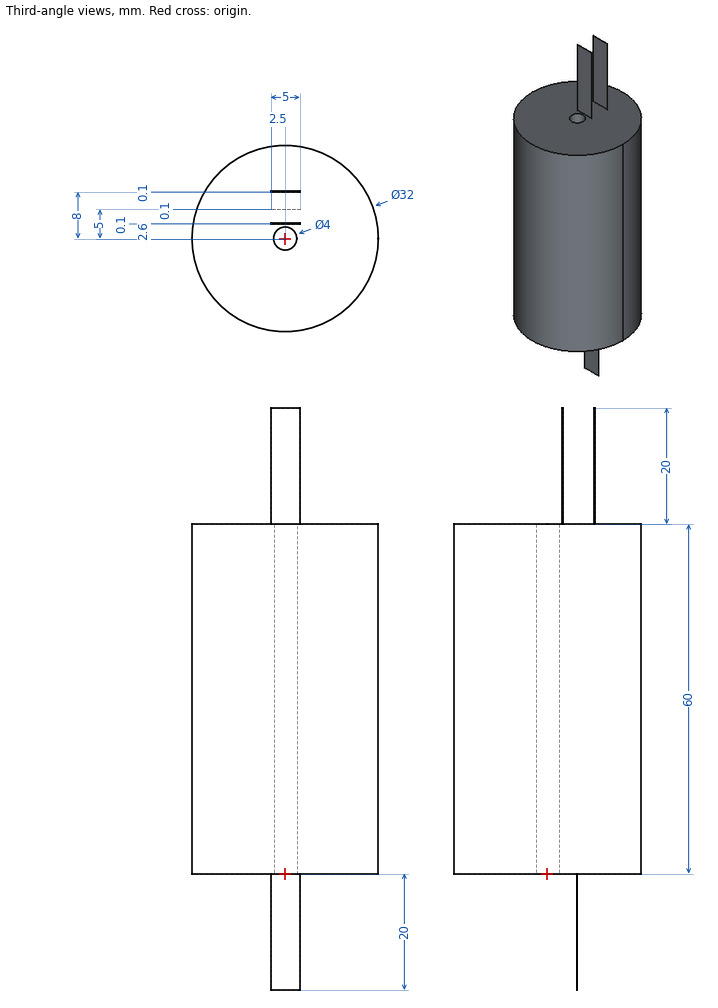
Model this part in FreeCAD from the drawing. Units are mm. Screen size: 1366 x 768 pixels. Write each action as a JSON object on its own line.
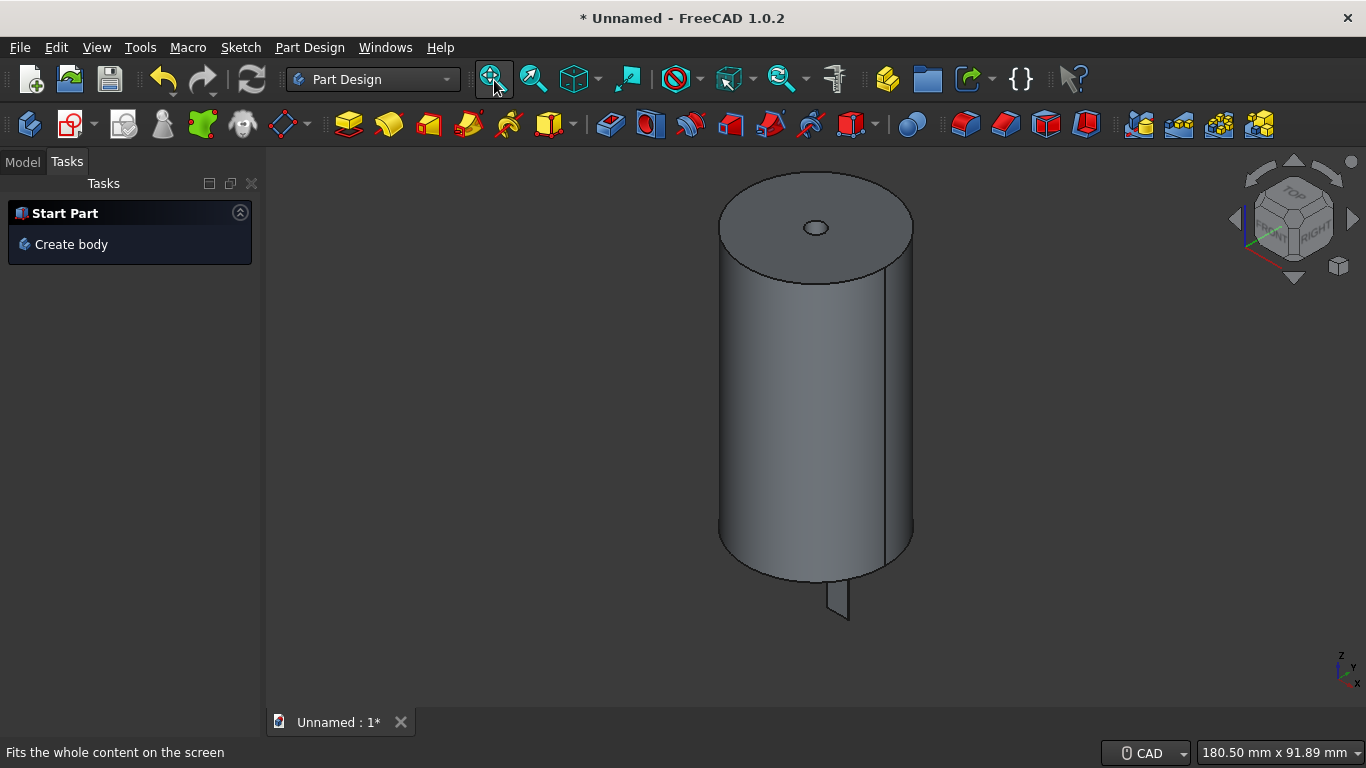
{"action": "left_click", "coordinate": [776, 250]}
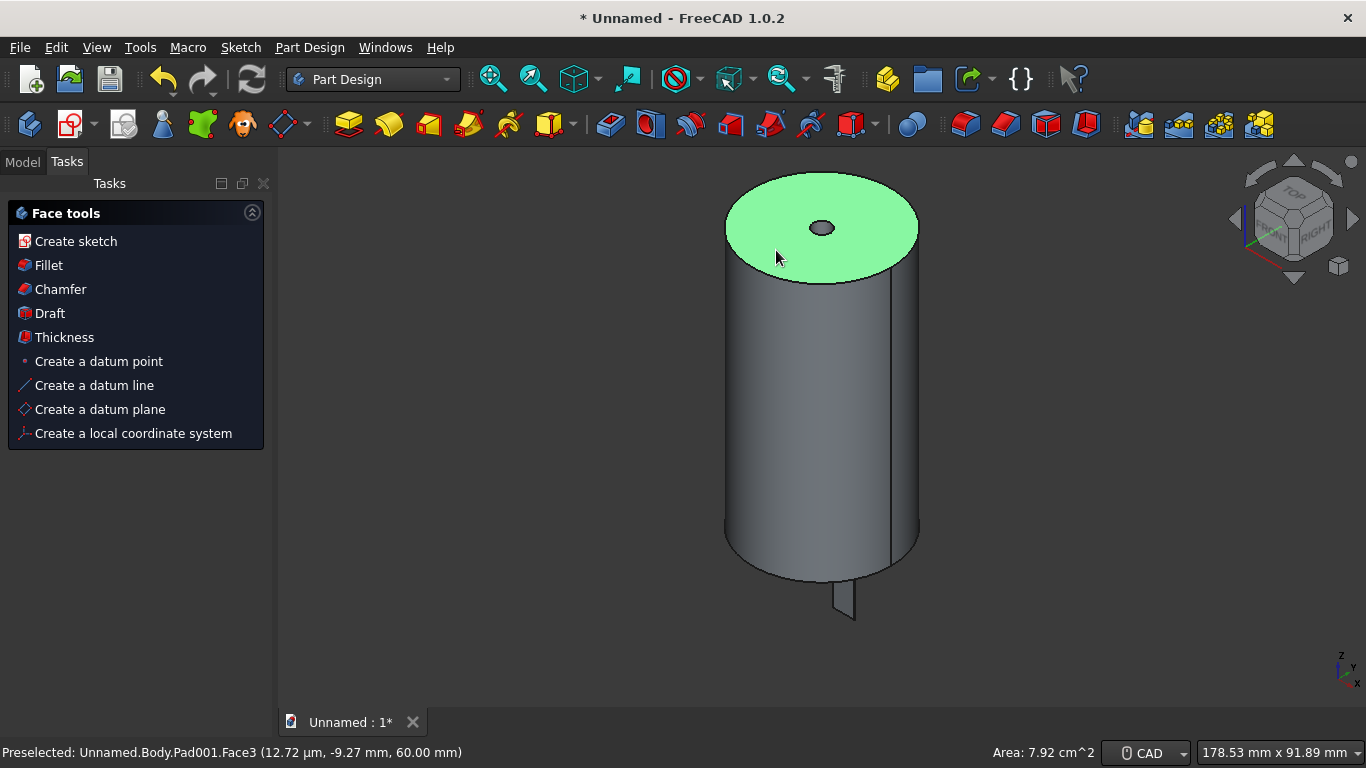
{"action": "left_click", "coordinate": [70, 124]}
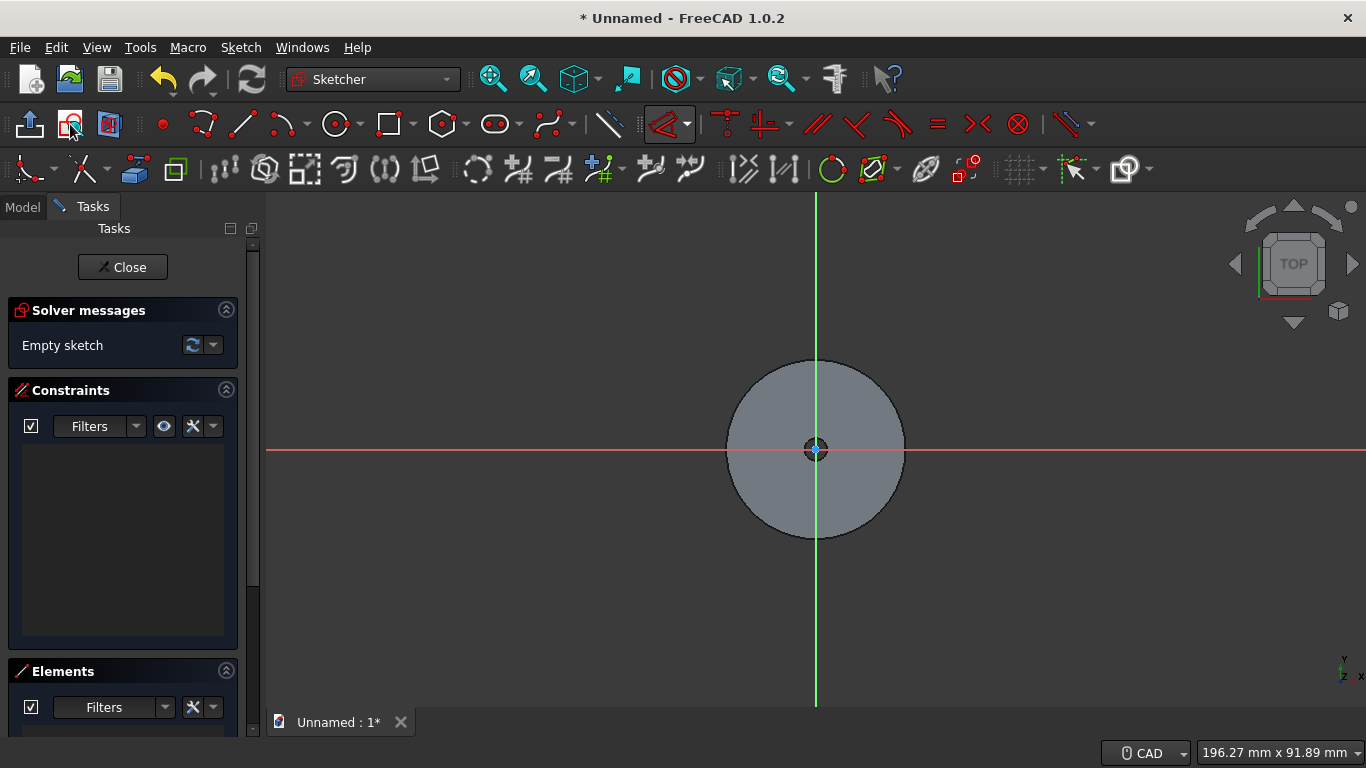
{"action": "scroll", "coordinate": [827, 423], "scroll_direction": "up", "scroll_amount": 10}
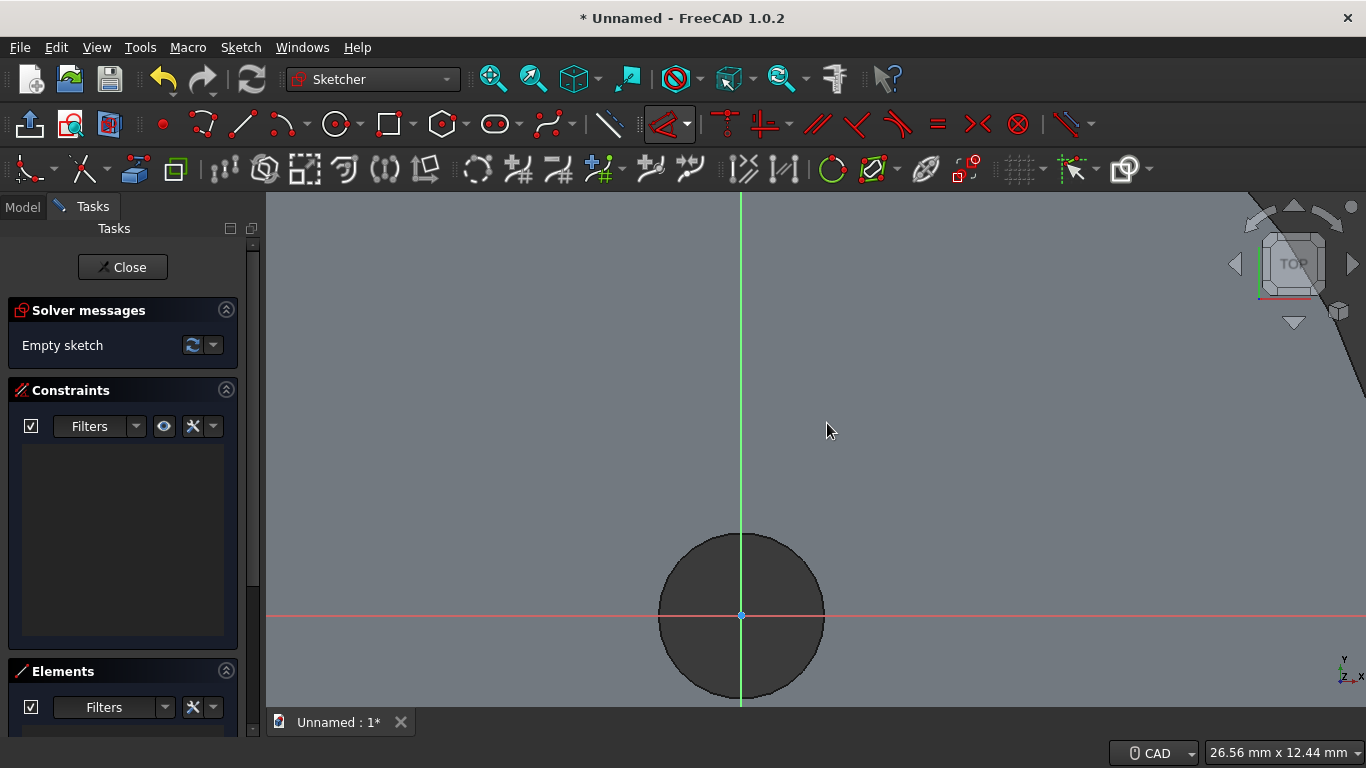
{"action": "left_click", "coordinate": [390, 124]}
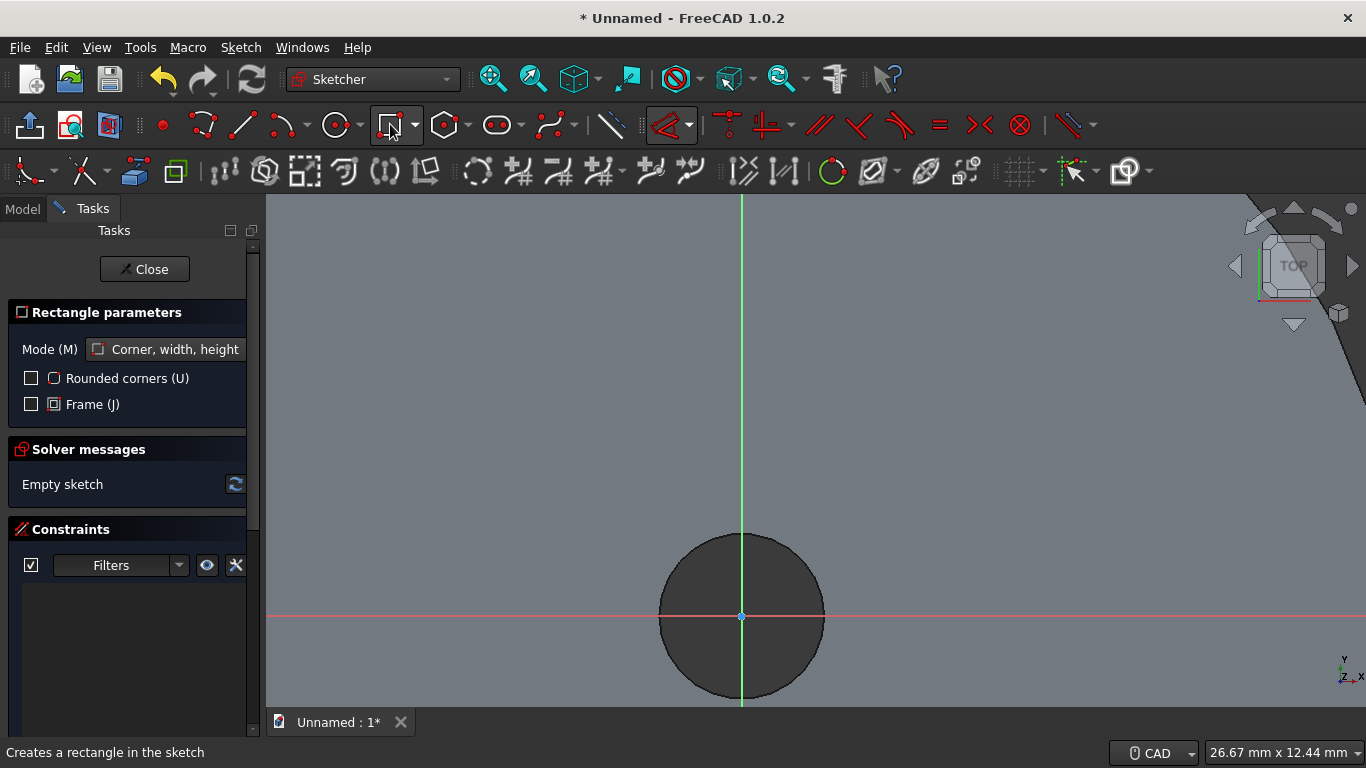
{"action": "scroll", "coordinate": [639, 282], "scroll_direction": "up", "scroll_amount": 7}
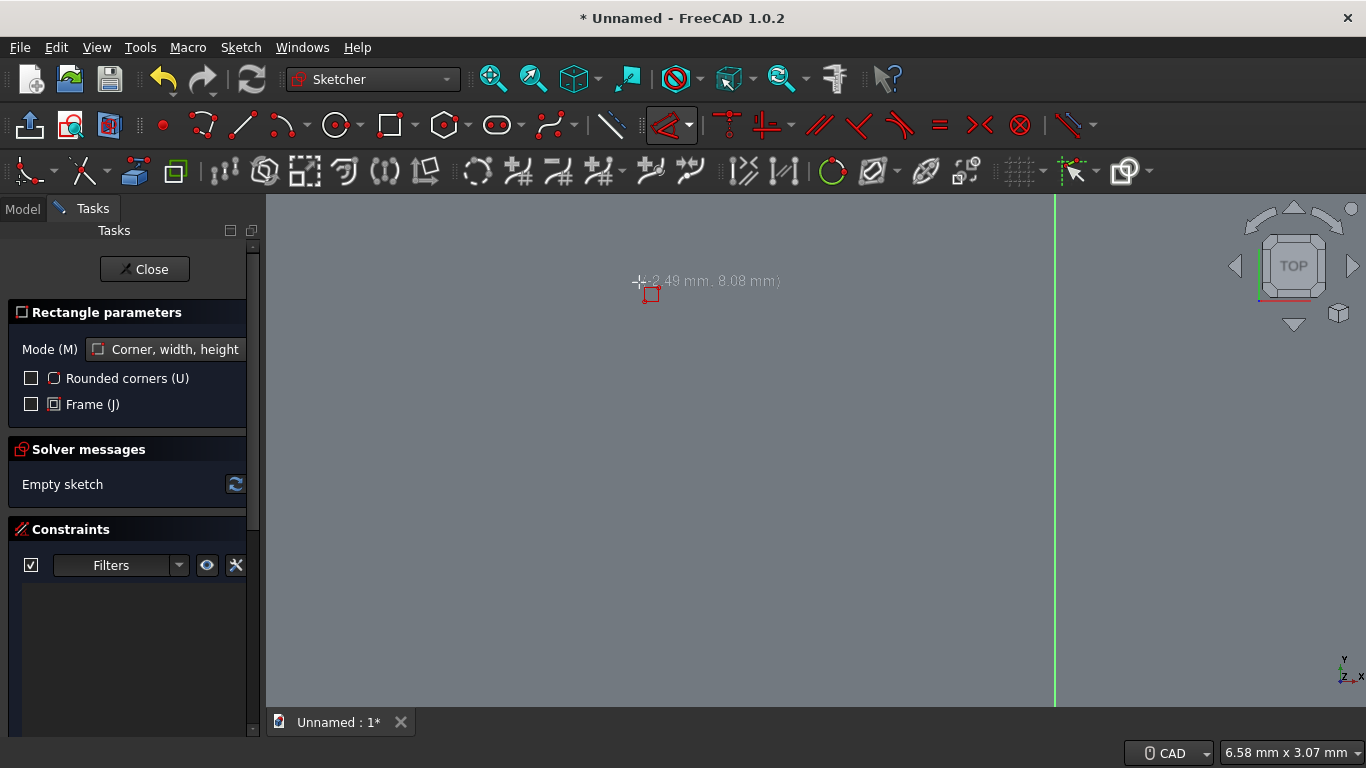
{"action": "scroll", "coordinate": [647, 284], "scroll_direction": "down", "scroll_amount": 7}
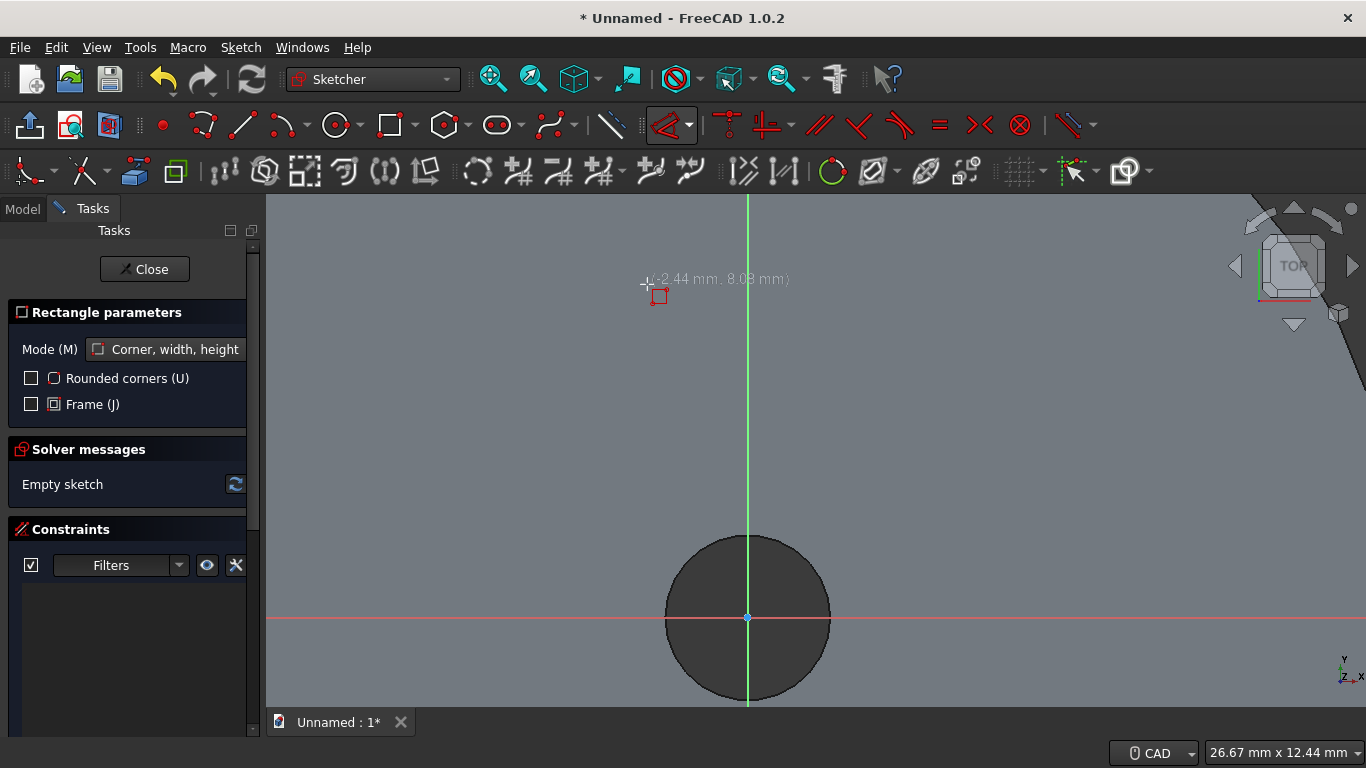
{"action": "left_click", "coordinate": [645, 284]}
{"action": "left_click", "coordinate": [851, 288]}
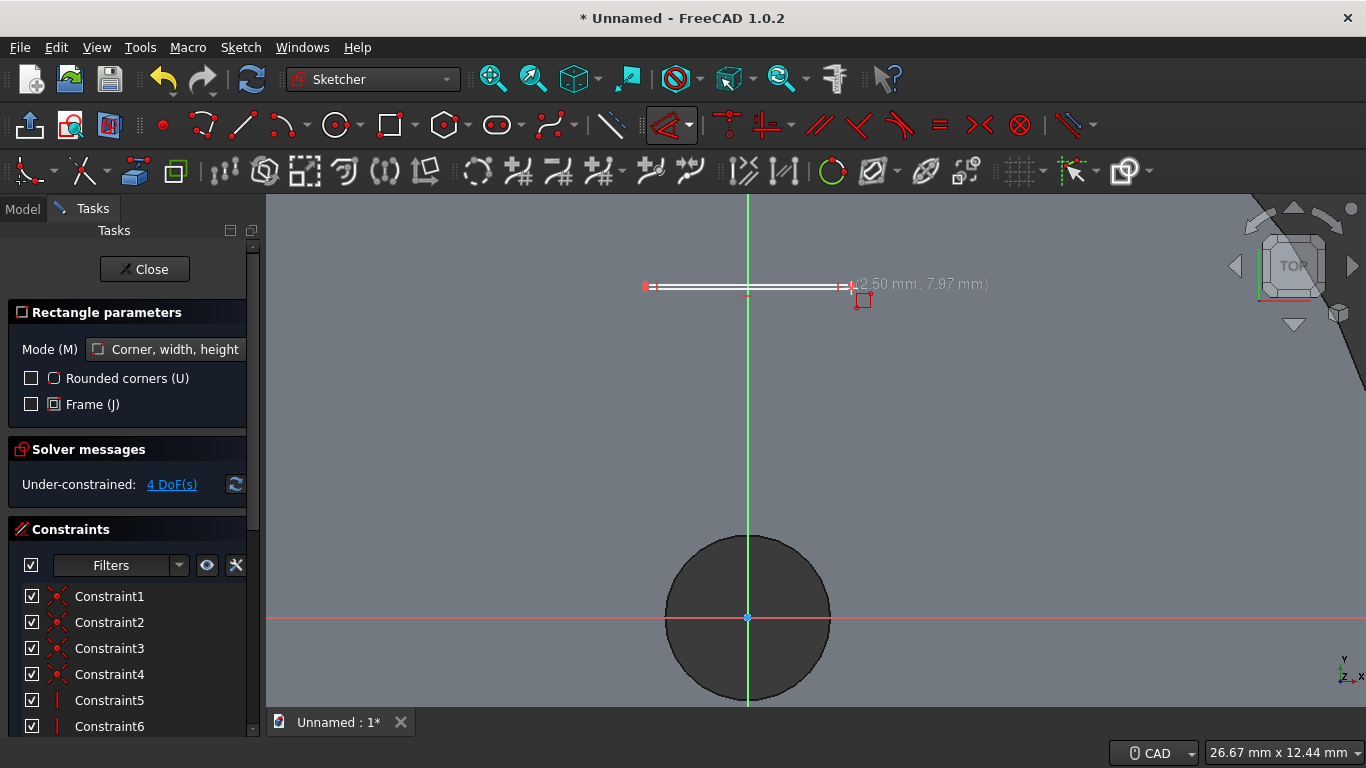
{"action": "scroll", "coordinate": [645, 511], "scroll_direction": "up", "scroll_amount": 7}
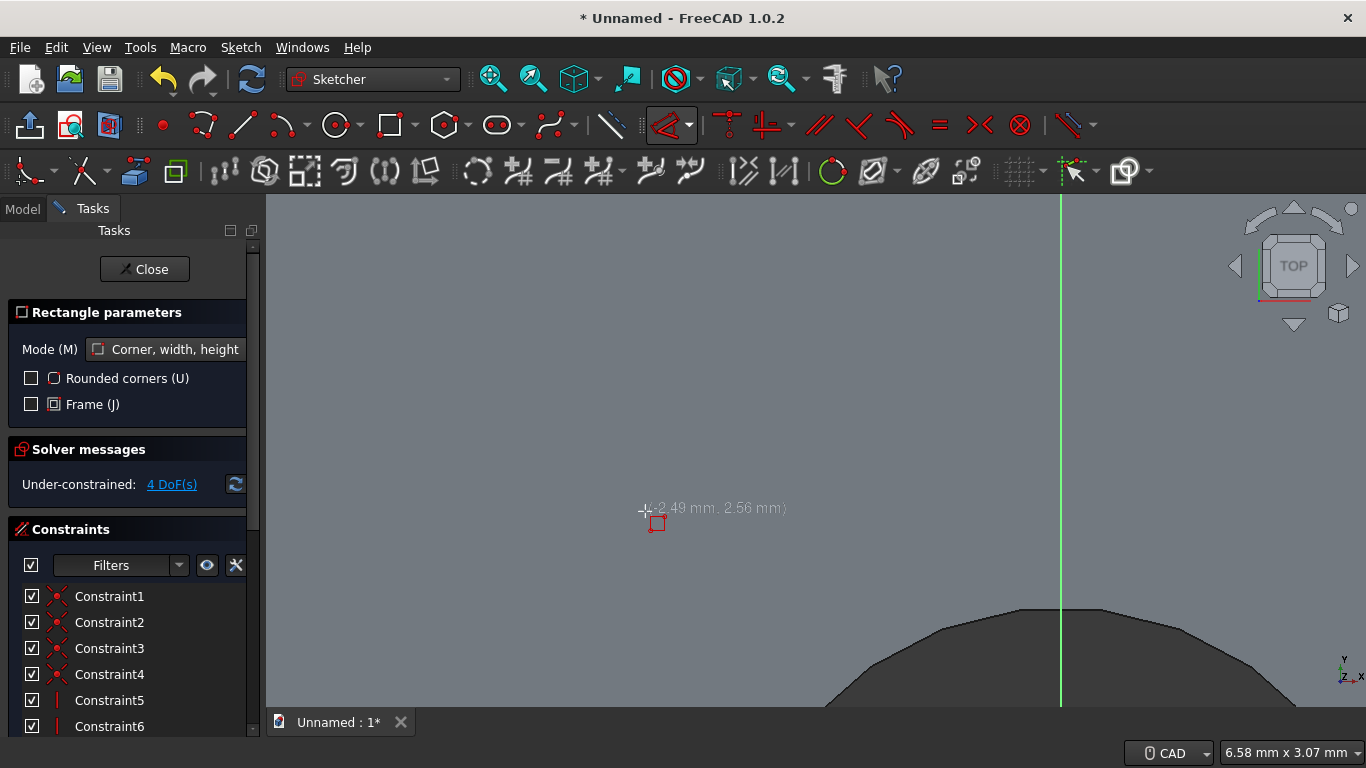
{"action": "scroll", "coordinate": [645, 511], "scroll_direction": "down", "scroll_amount": 7}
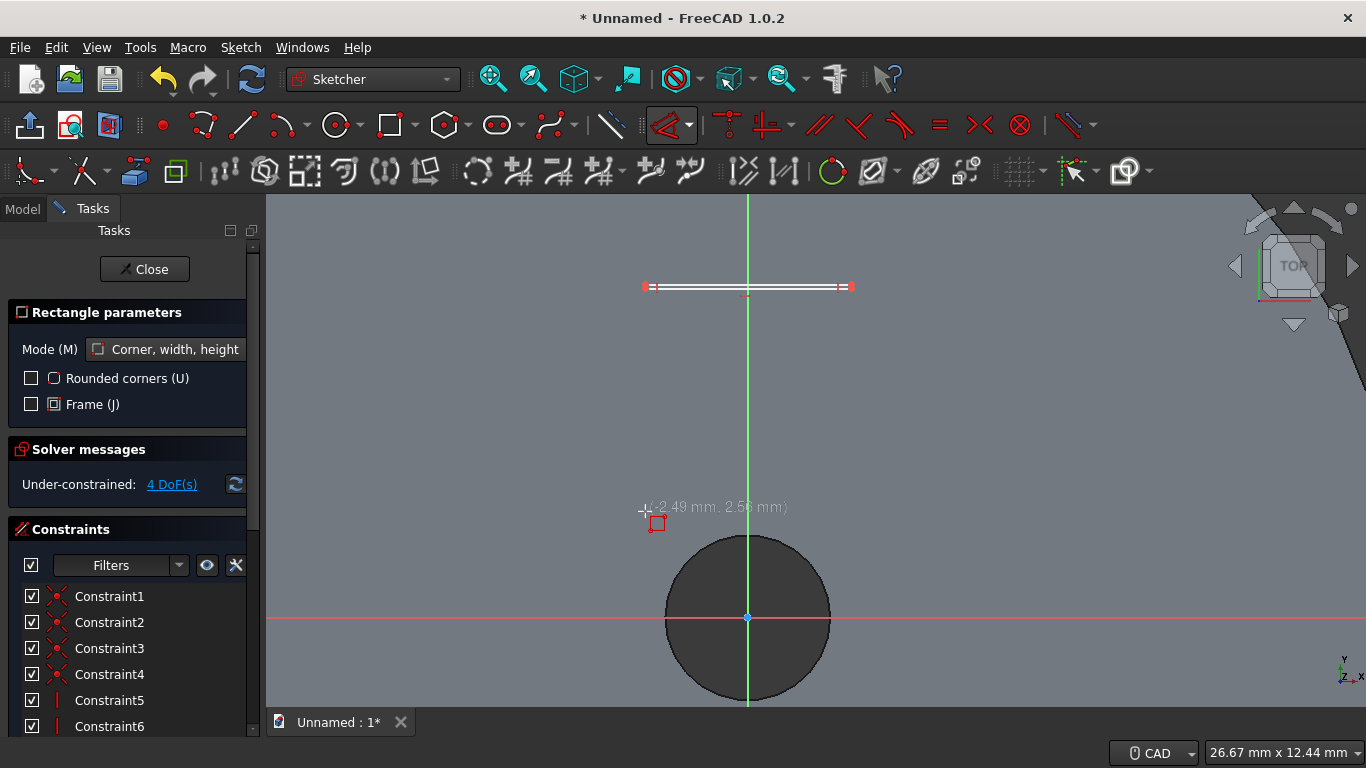
{"action": "left_click", "coordinate": [645, 511]}
{"action": "left_click", "coordinate": [851, 515]}
{"action": "key", "text": "Escape"}